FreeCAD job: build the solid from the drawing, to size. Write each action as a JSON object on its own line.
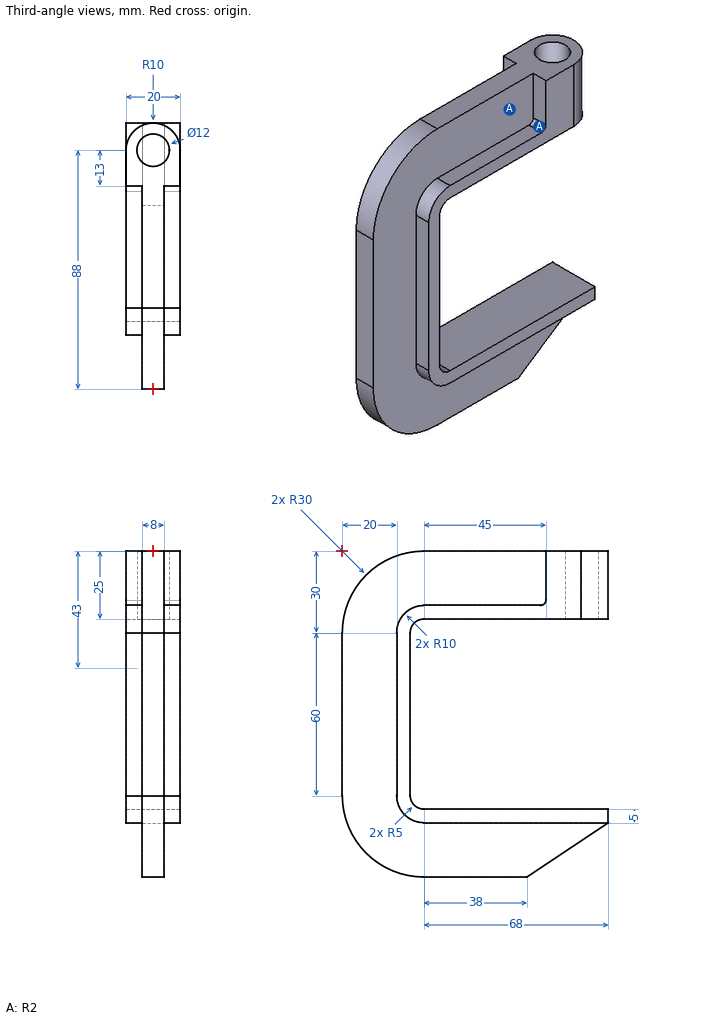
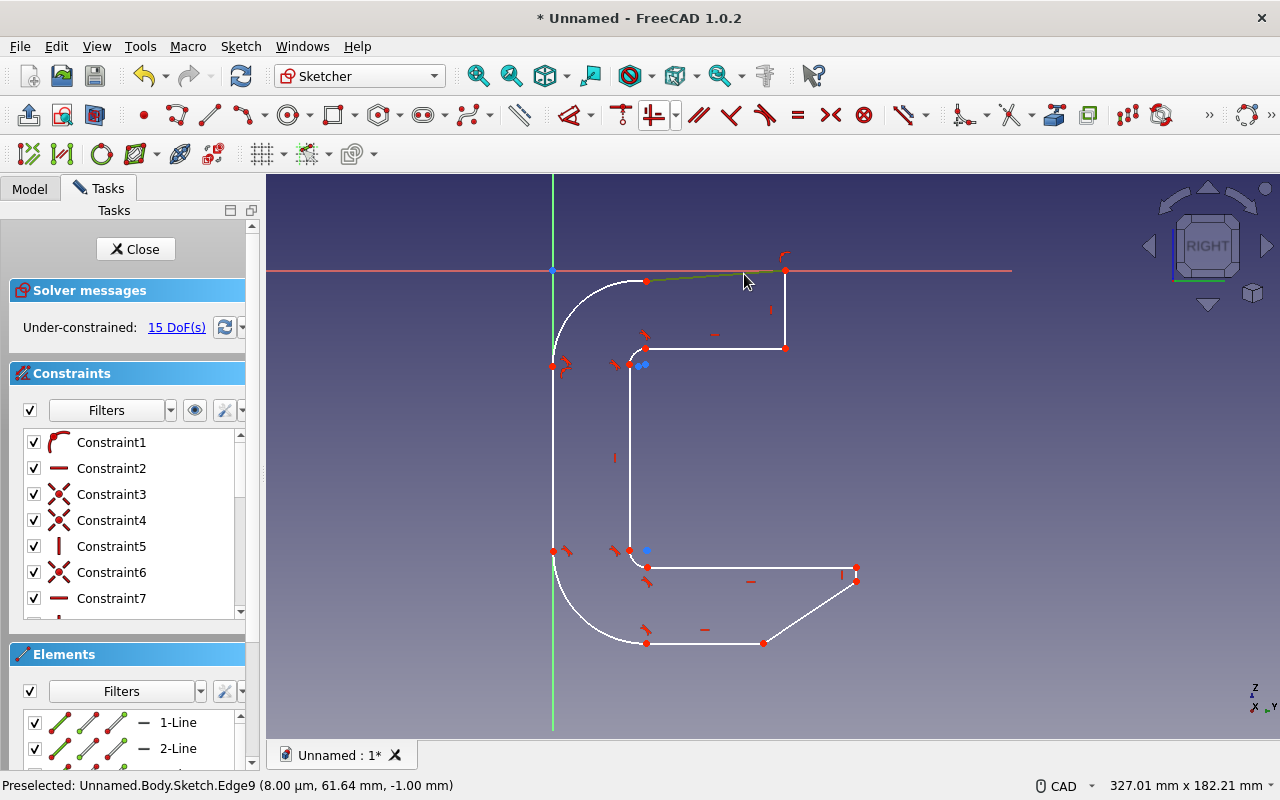
{"action": "left_click", "coordinate": [604, 288]}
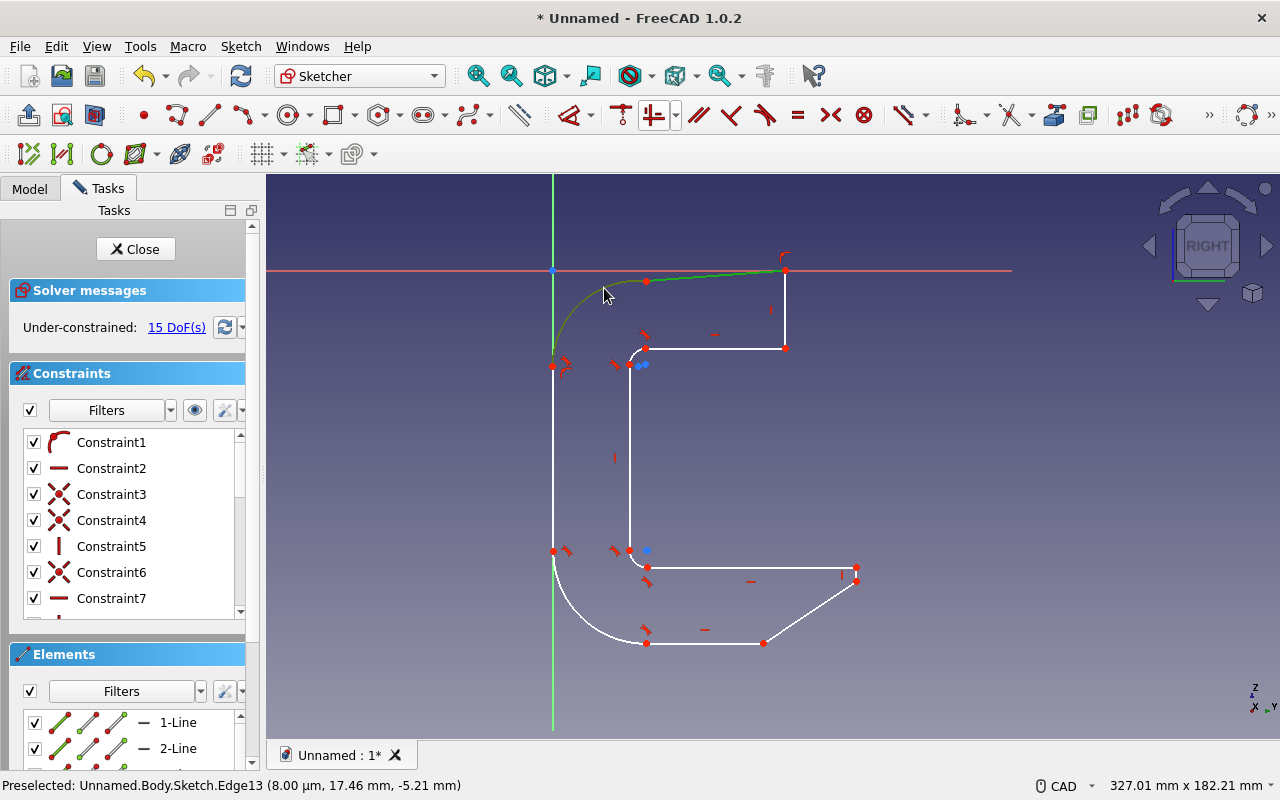
{"action": "left_click", "coordinate": [765, 116]}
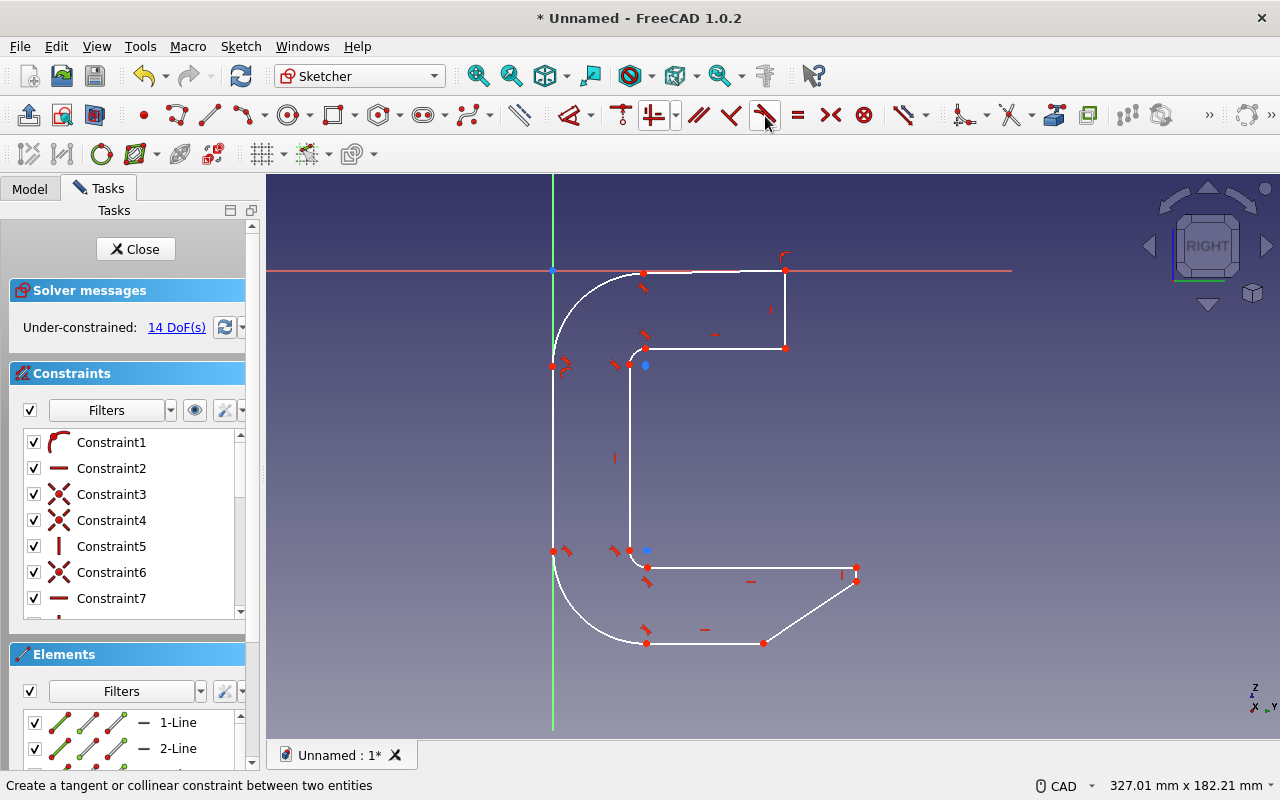
{"action": "left_click", "coordinate": [553, 422]}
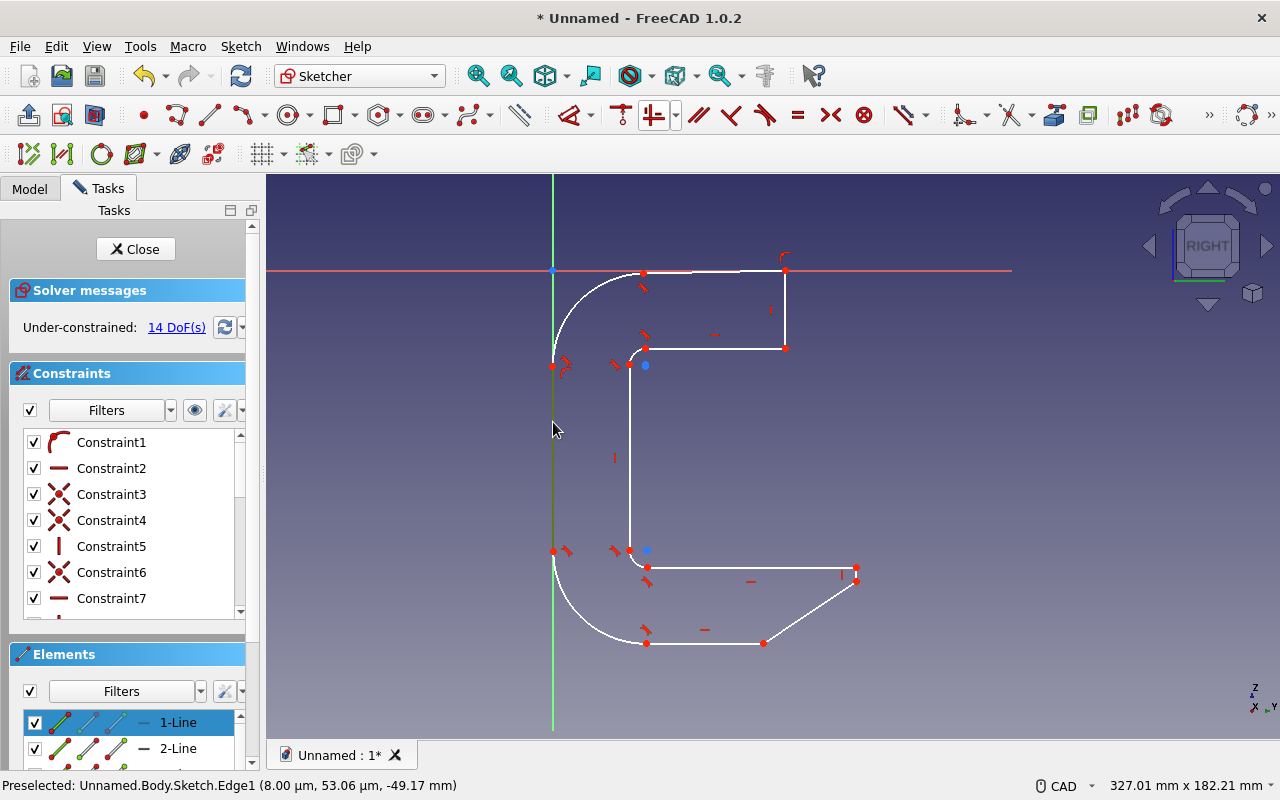
{"action": "key", "text": "v"}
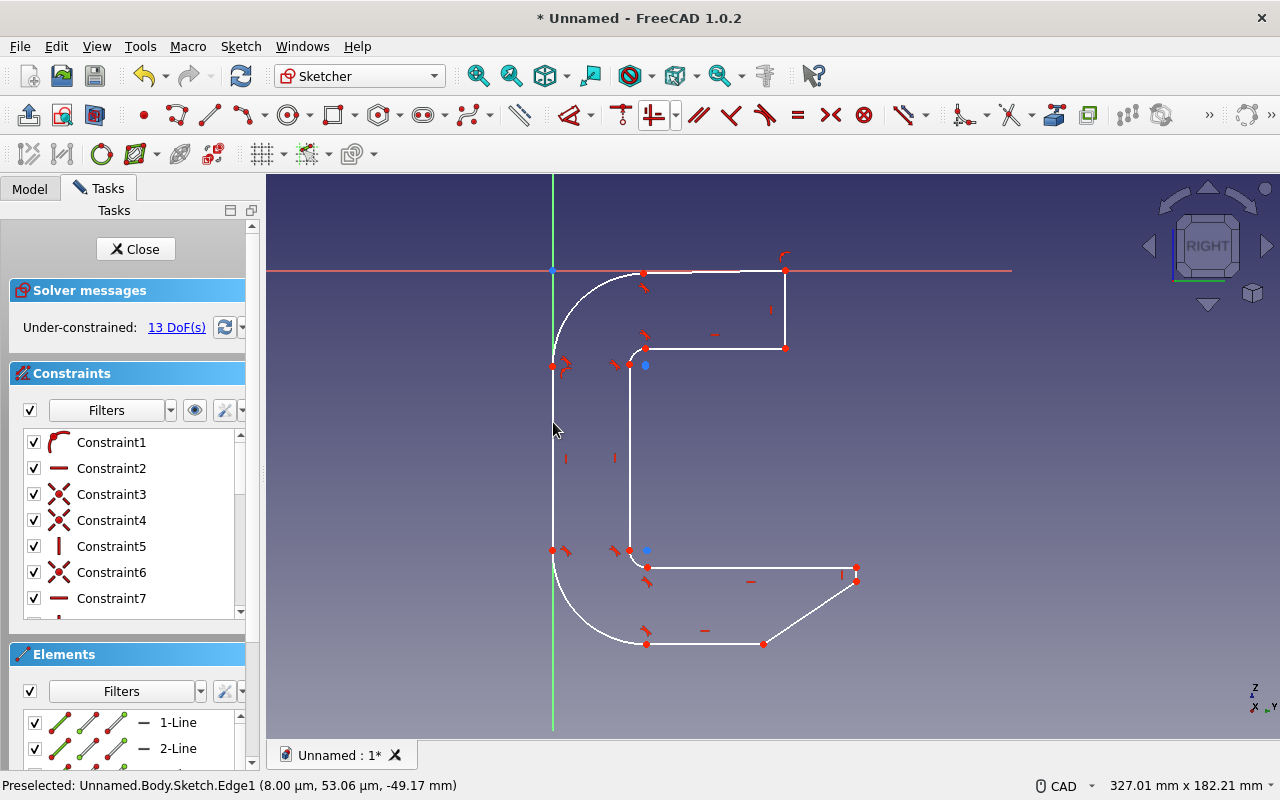
{"action": "left_click", "coordinate": [743, 271]}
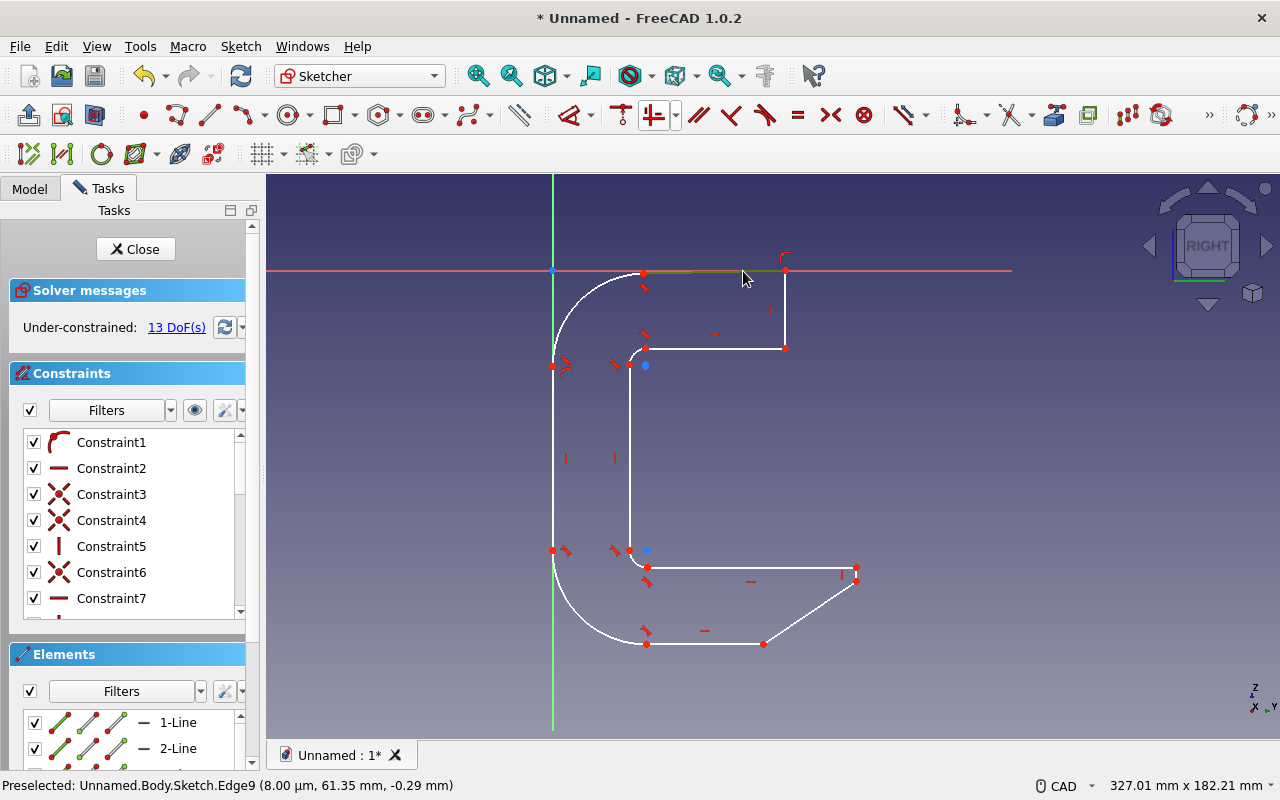
{"action": "key", "text": "h"}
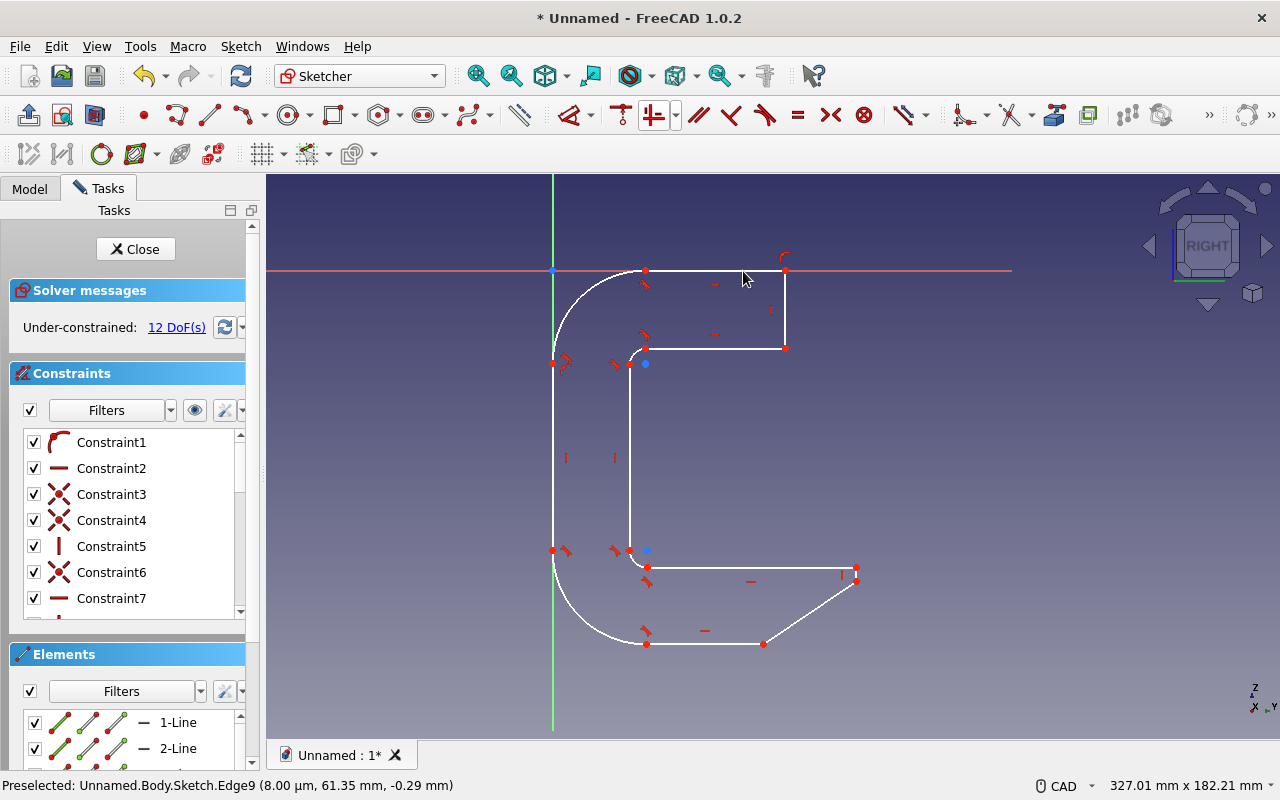
{"action": "scroll", "coordinate": [563, 593], "scroll_direction": "up", "scroll_amount": 2}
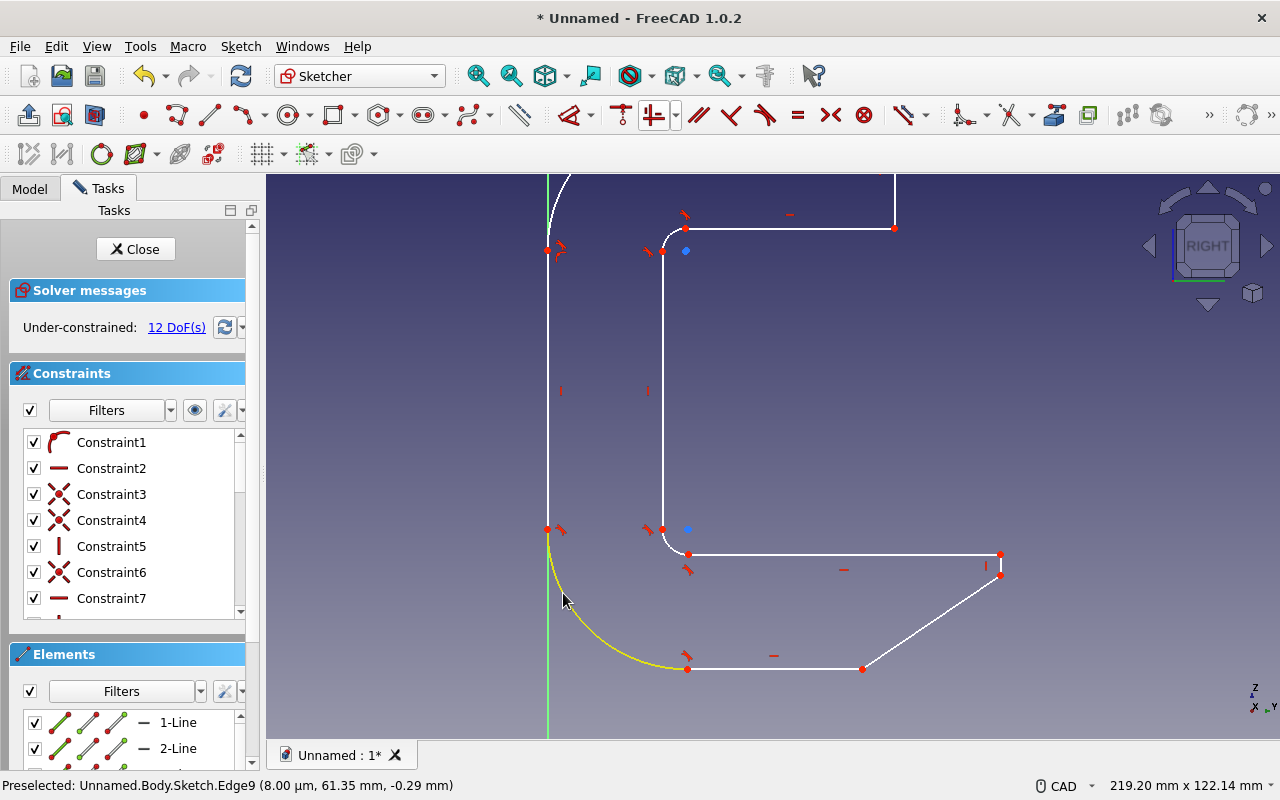
{"action": "left_click", "coordinate": [563, 593]}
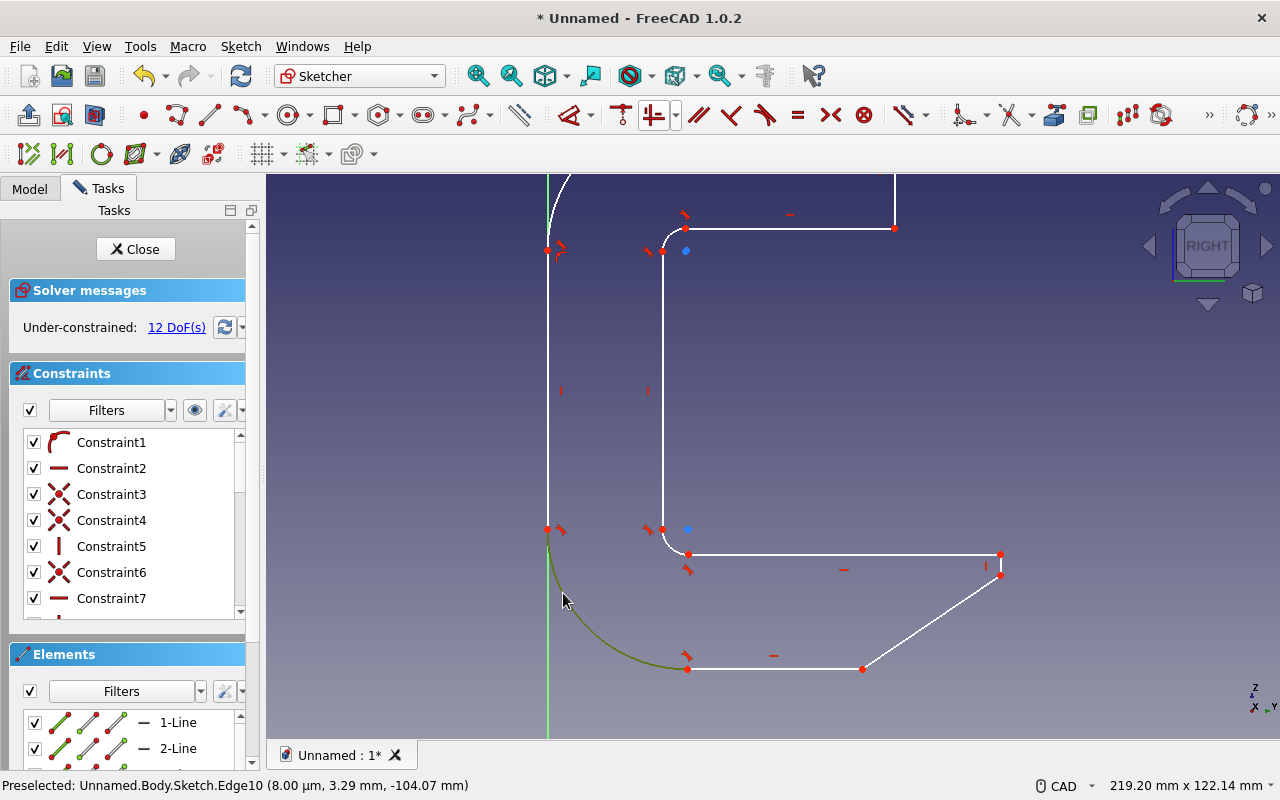
{"action": "left_click", "coordinate": [665, 541]}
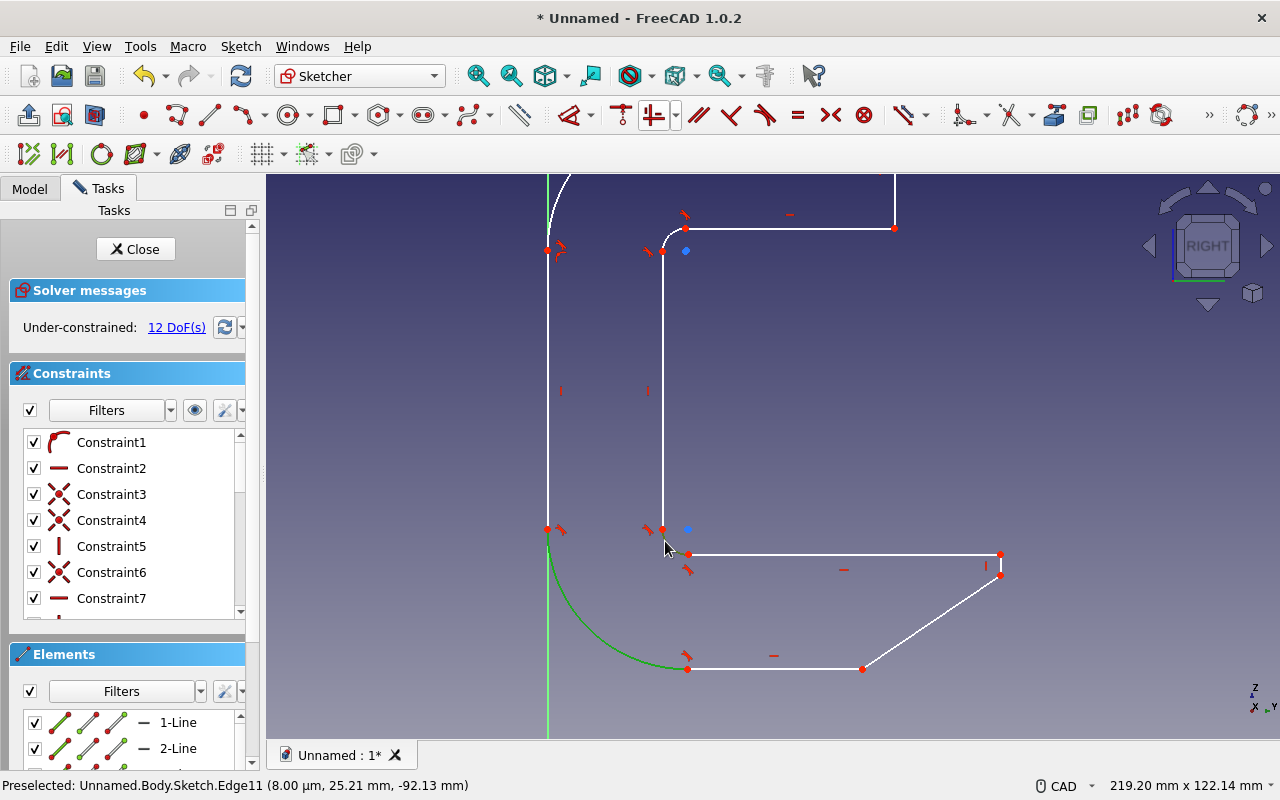
{"action": "key", "text": "c"}